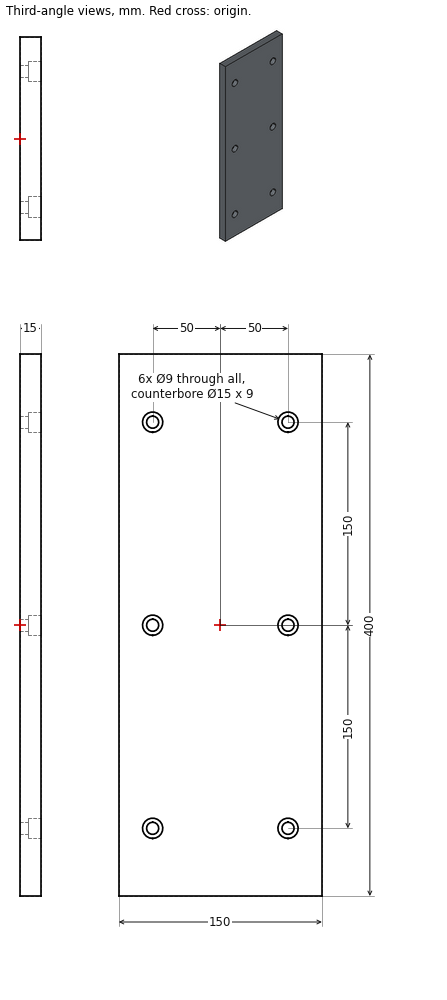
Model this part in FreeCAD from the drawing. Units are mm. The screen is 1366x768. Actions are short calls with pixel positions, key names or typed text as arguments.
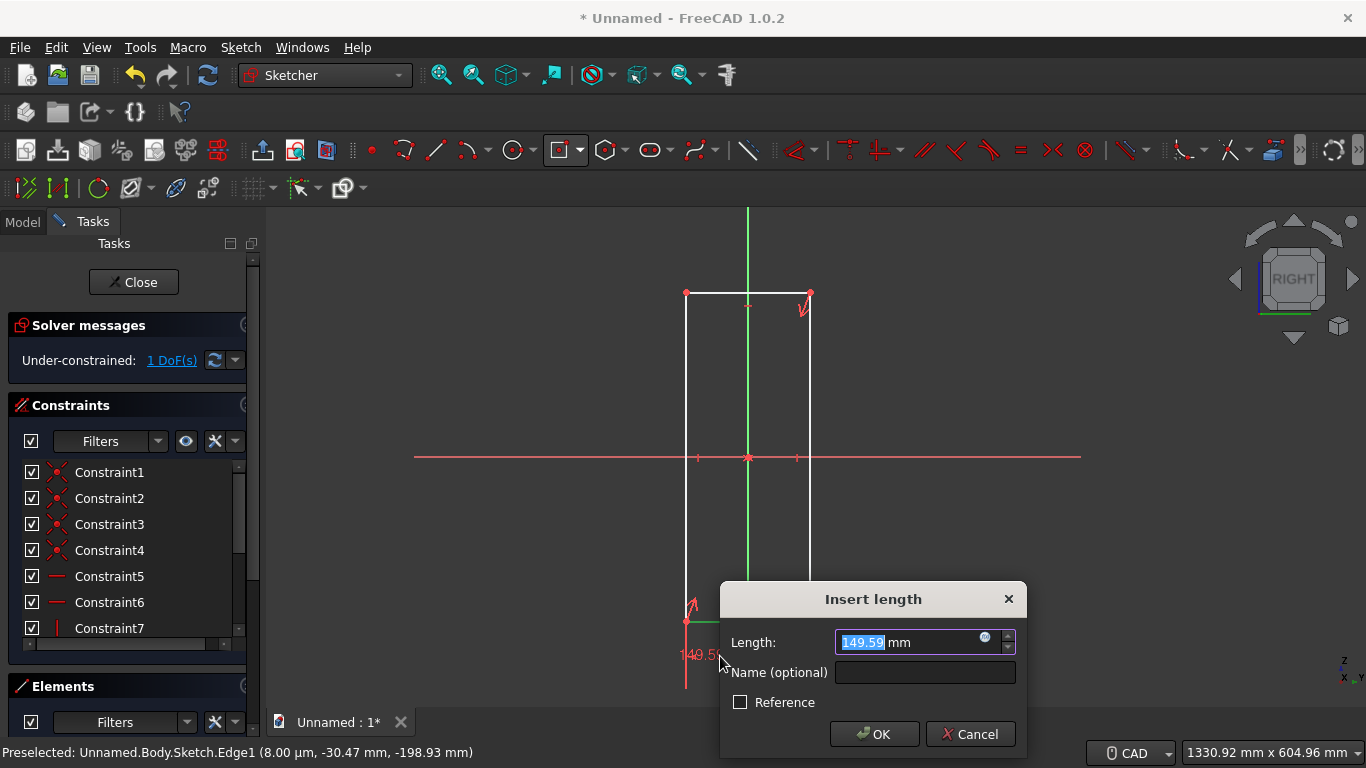
text(150)
key(Return)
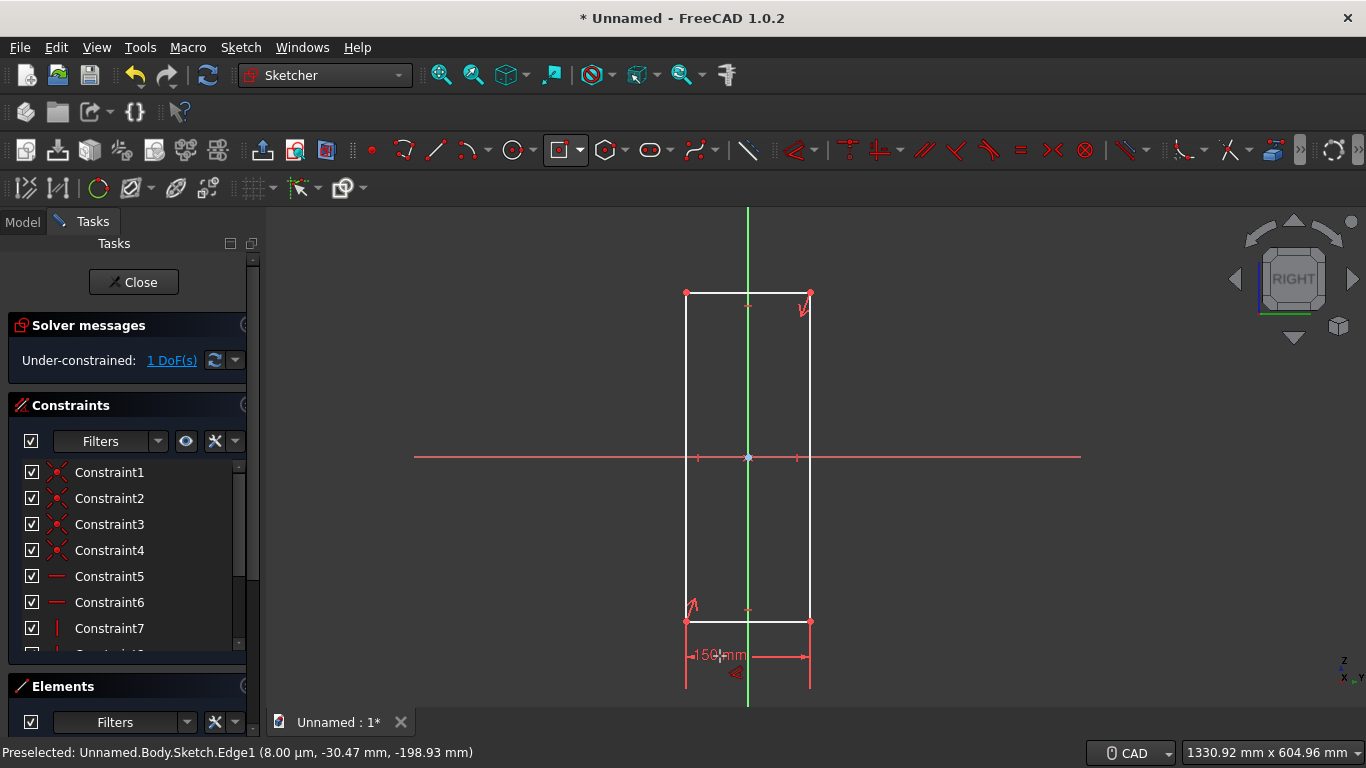
click(810, 523)
click(844, 382)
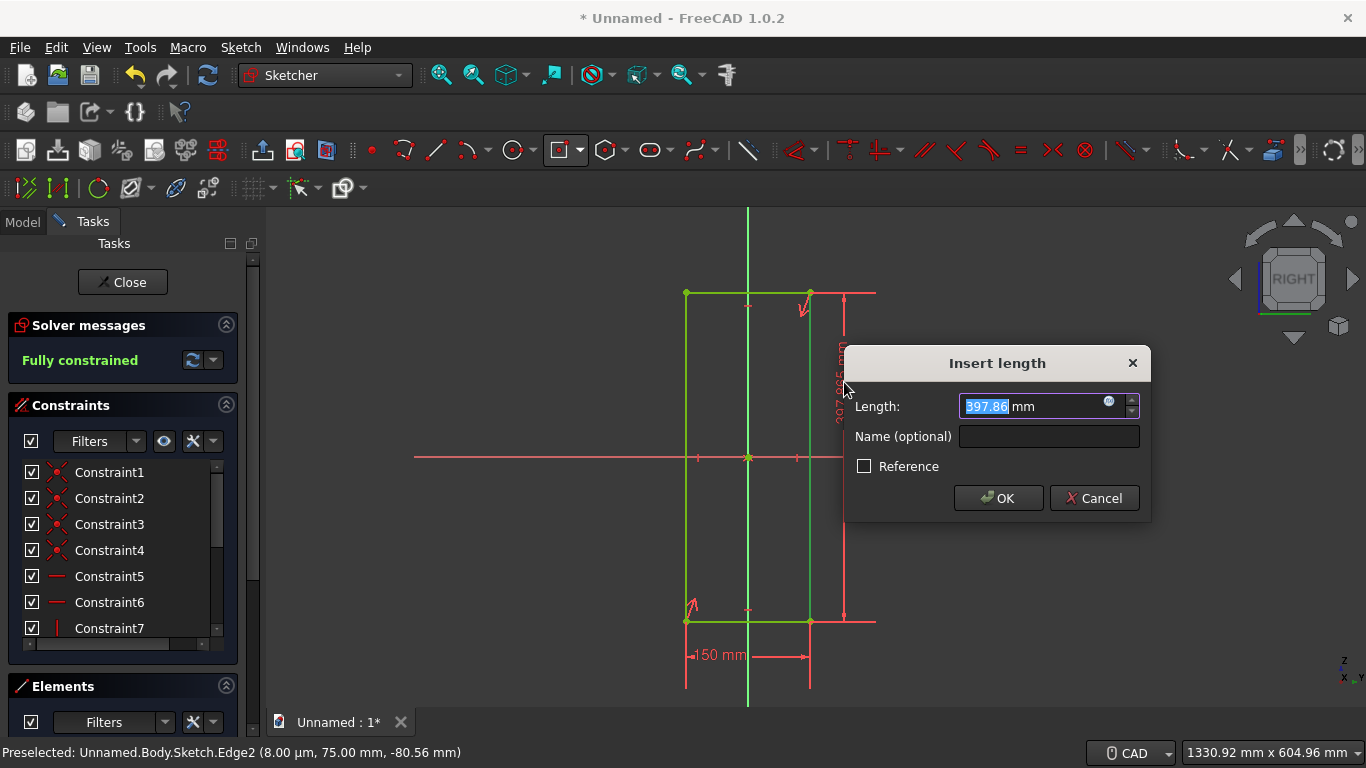
text(400)
key(Return)
key(Escape)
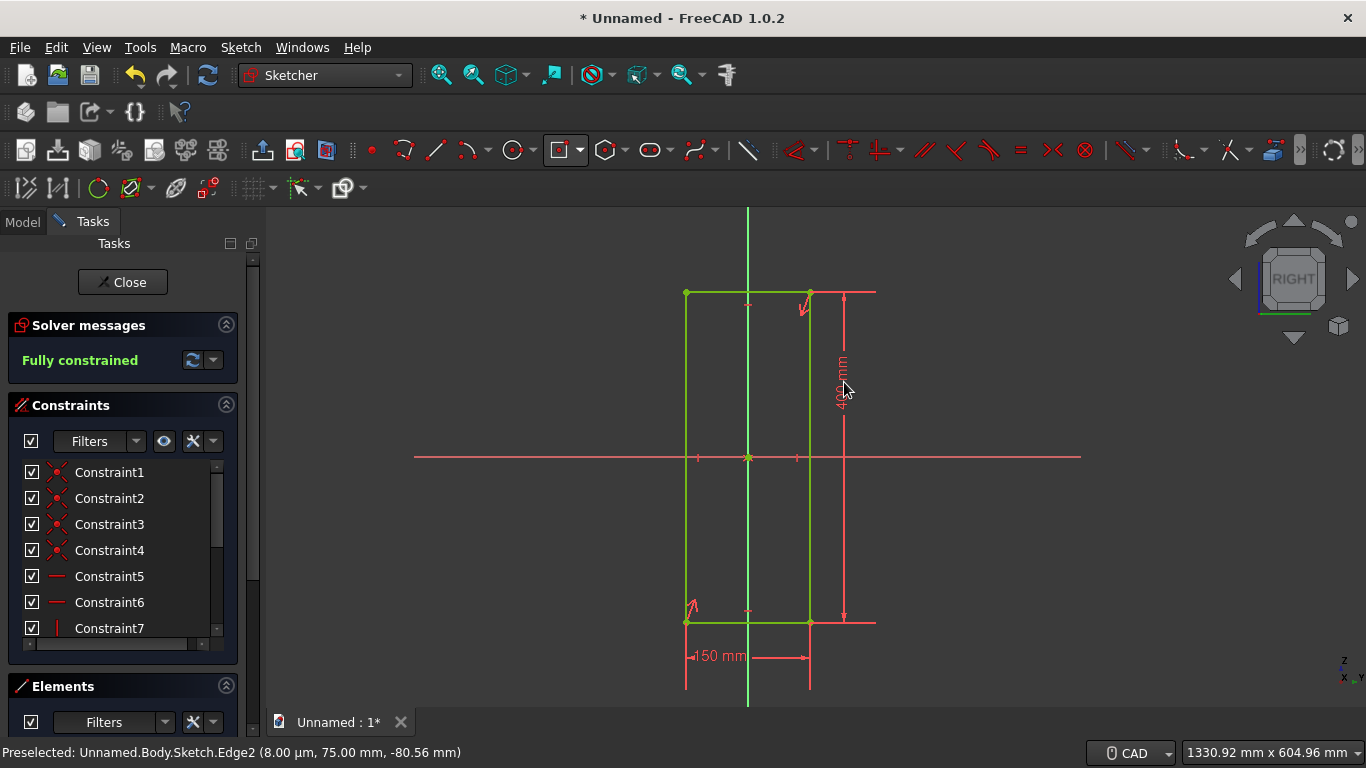
click(123, 282)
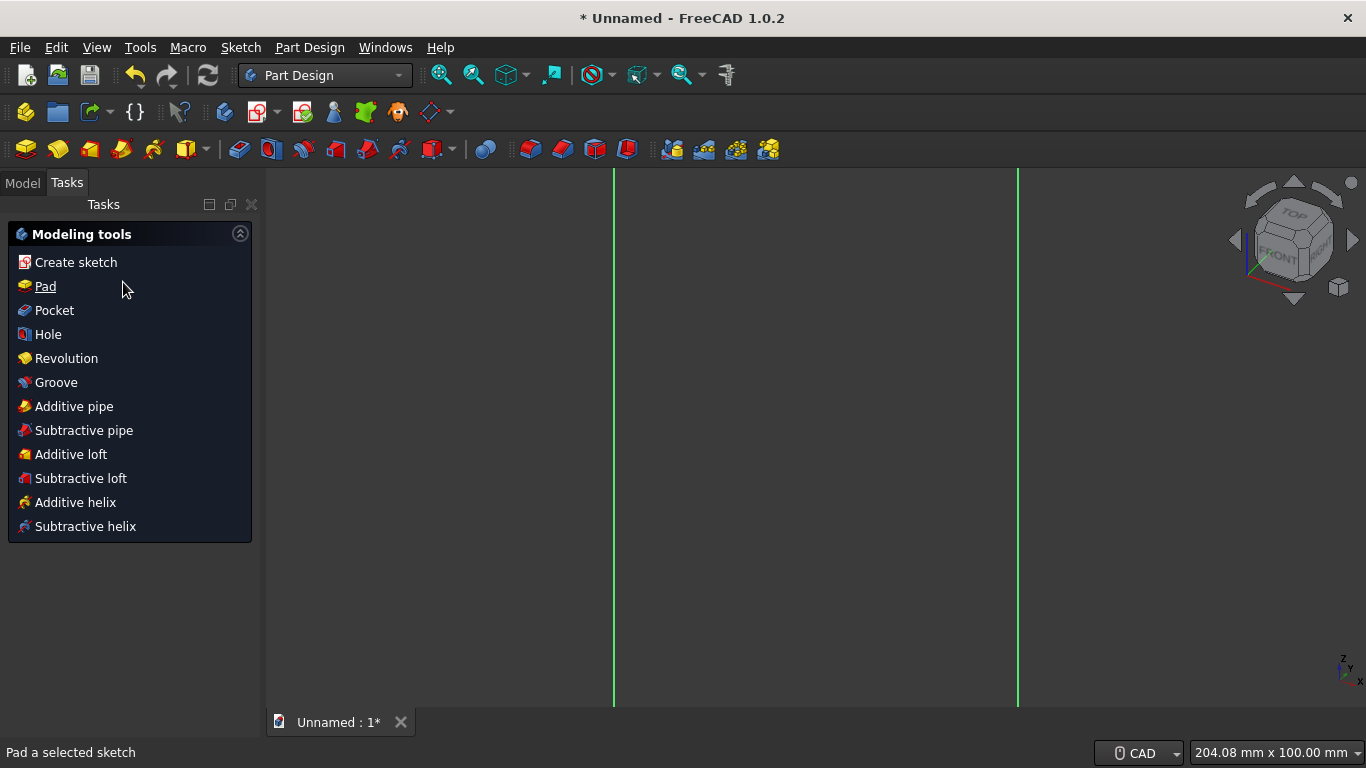
click(26, 150)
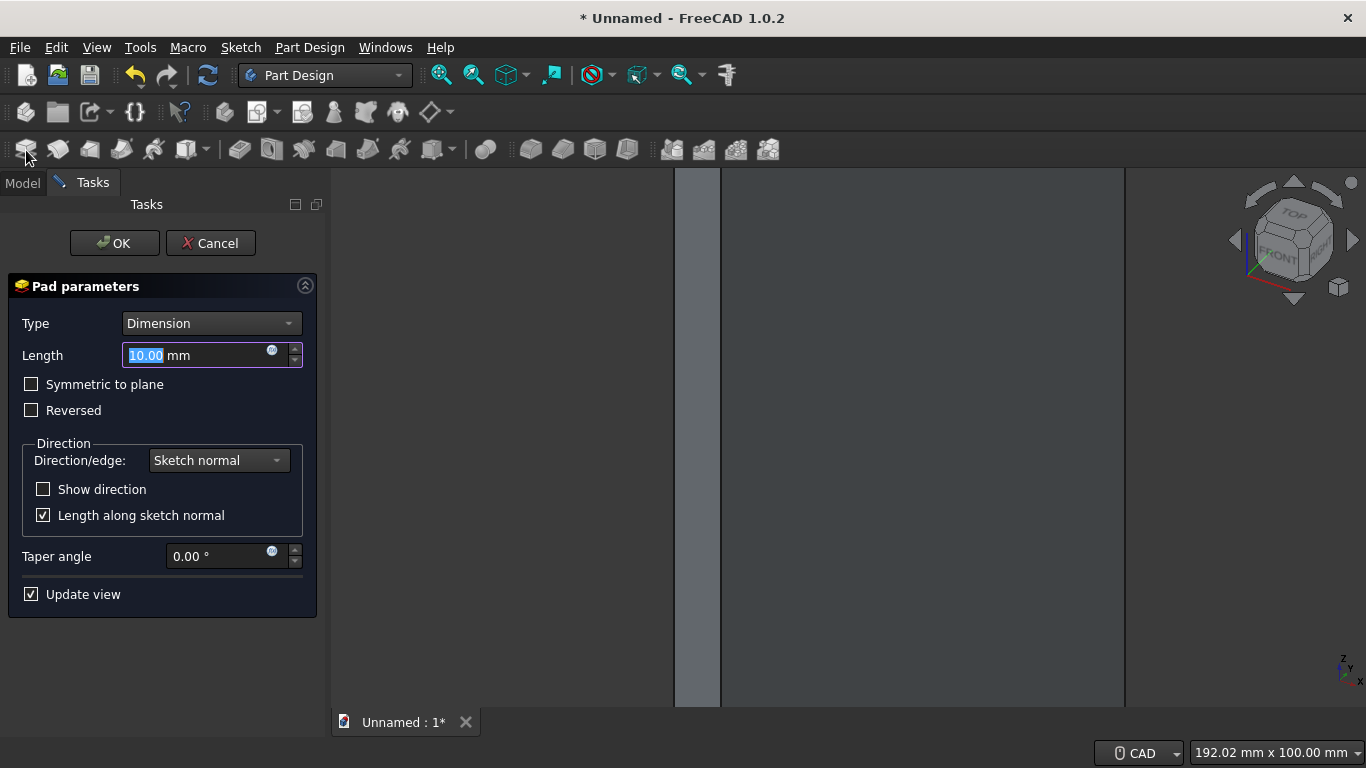
text(15)
key(Tab)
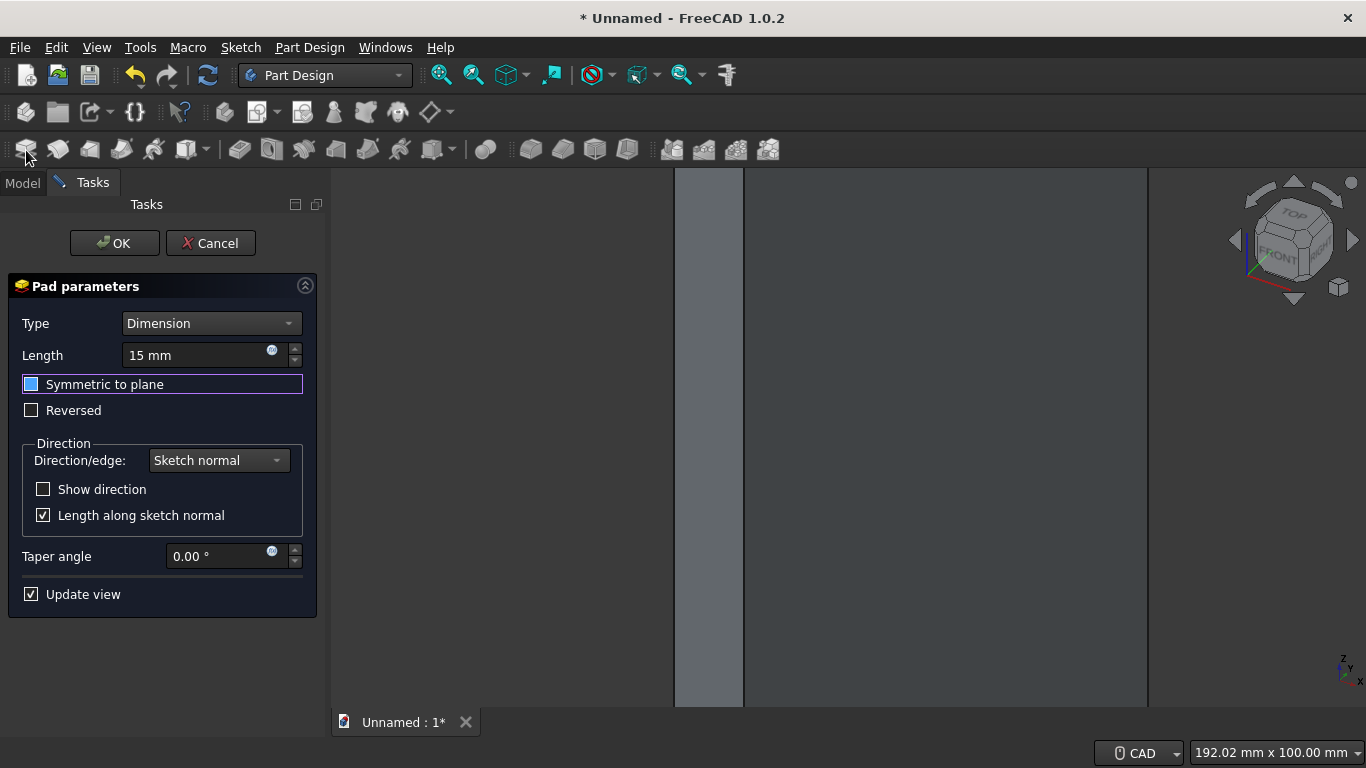
click(115, 243)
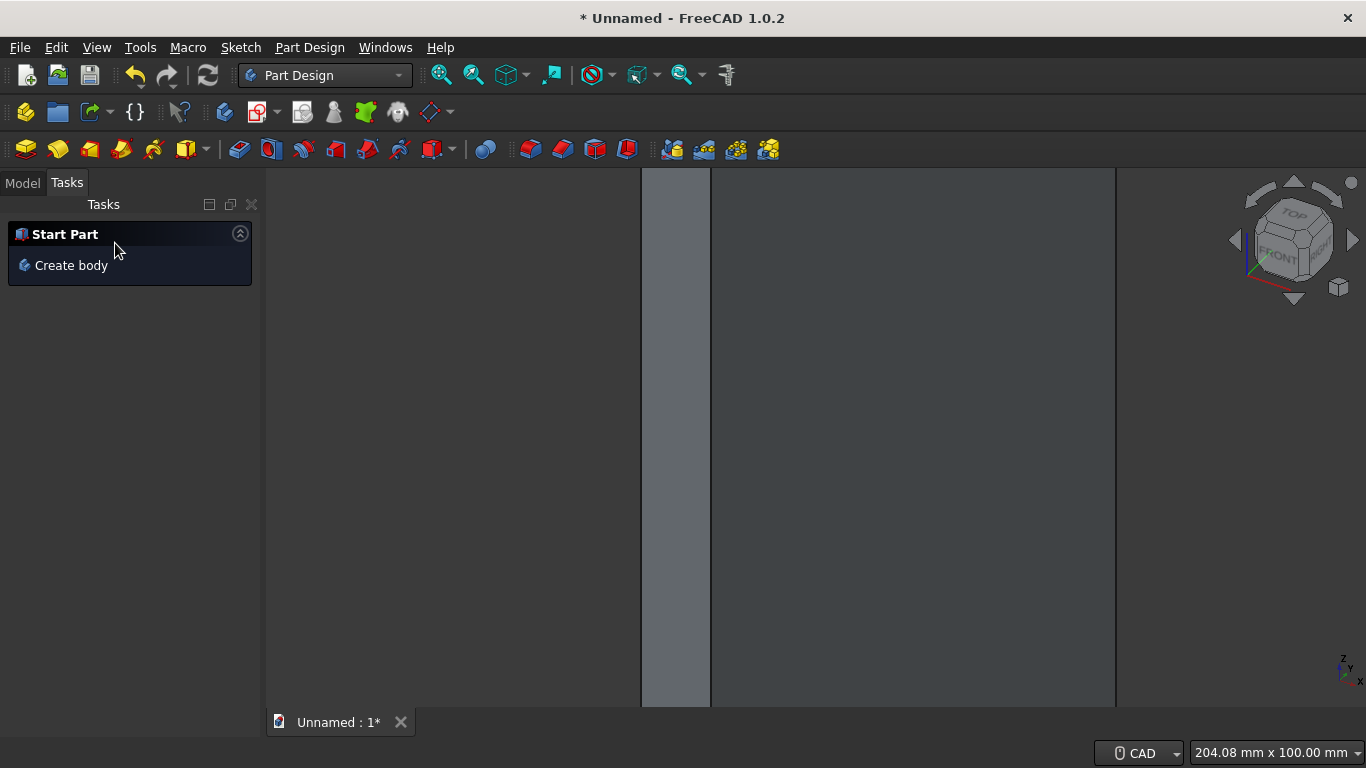
key(v)
key(f)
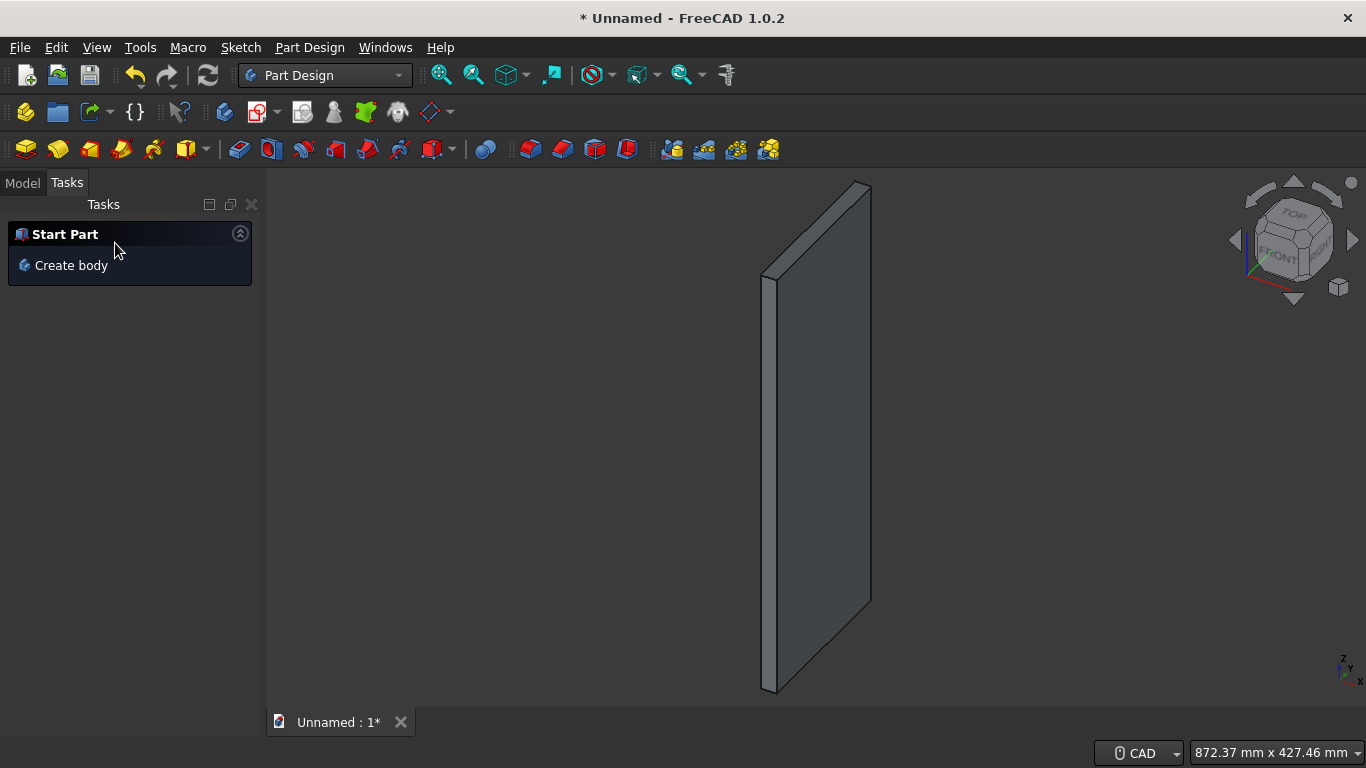
click(824, 439)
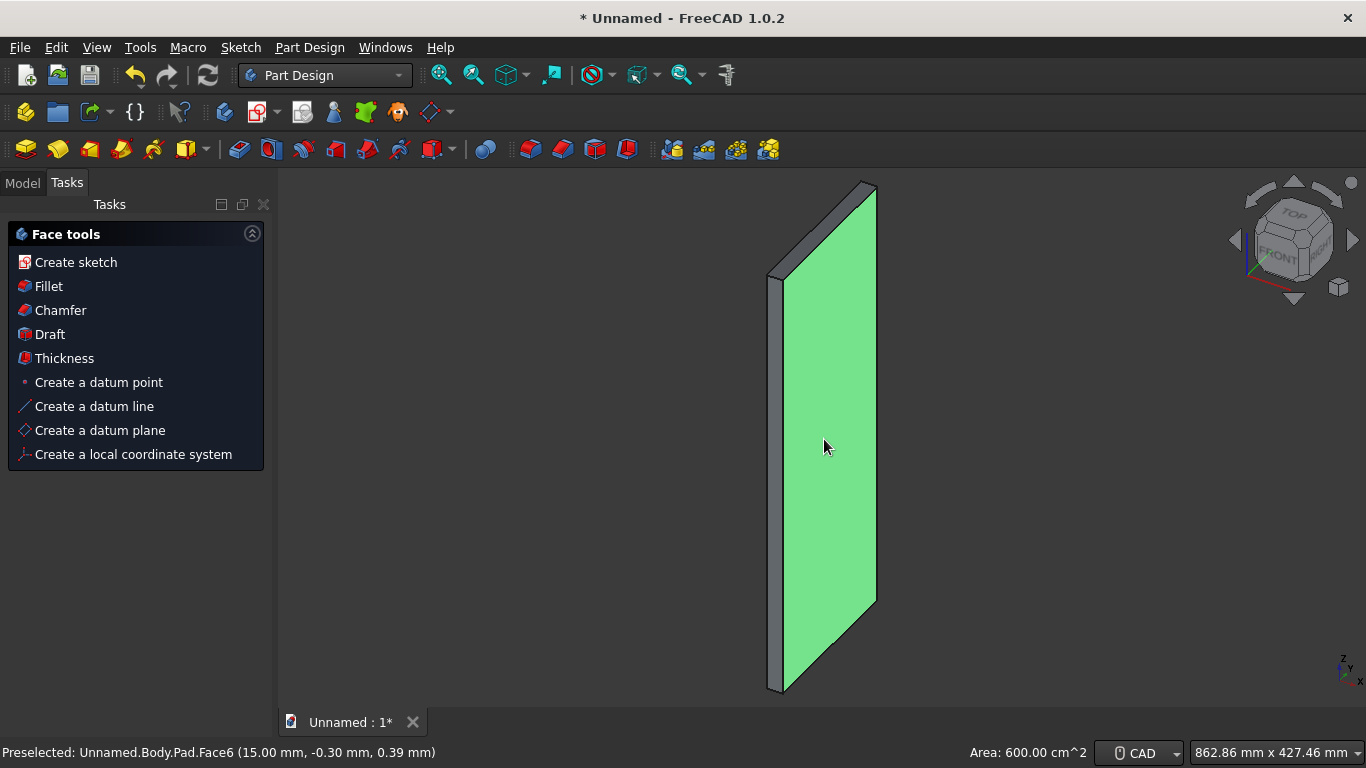
click(258, 112)